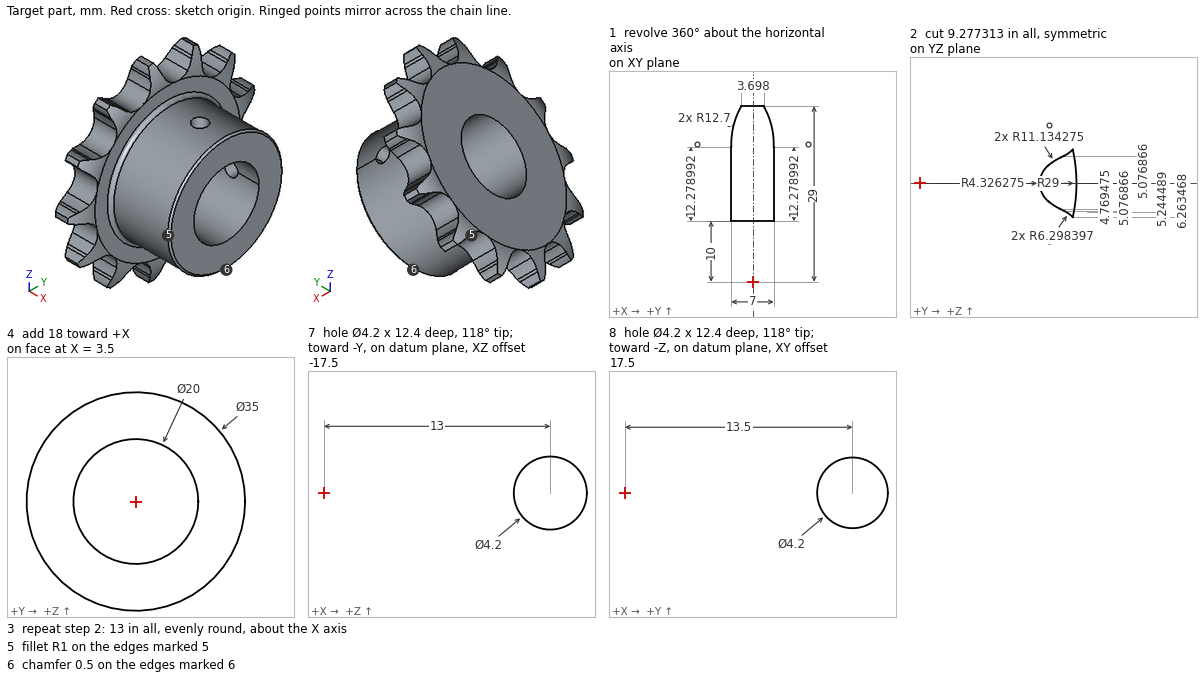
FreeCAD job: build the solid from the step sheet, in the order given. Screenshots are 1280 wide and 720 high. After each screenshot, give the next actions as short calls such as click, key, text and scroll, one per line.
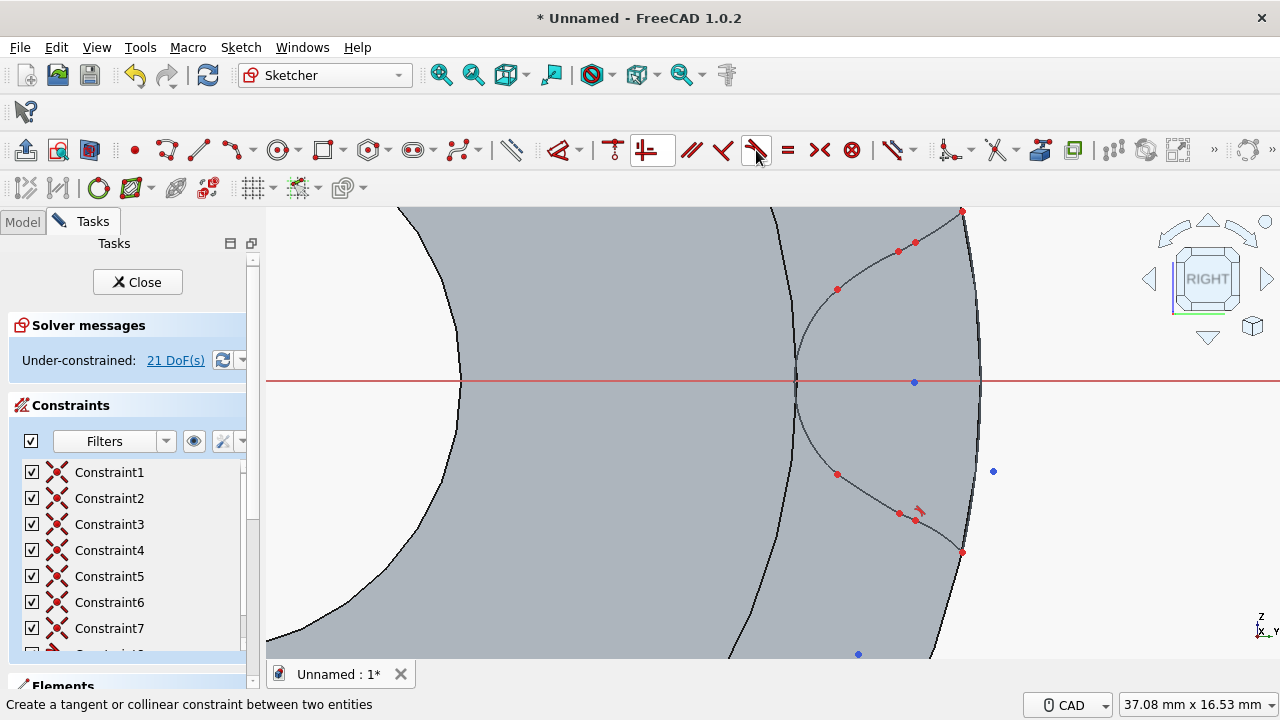
scroll(908, 517, up, 3)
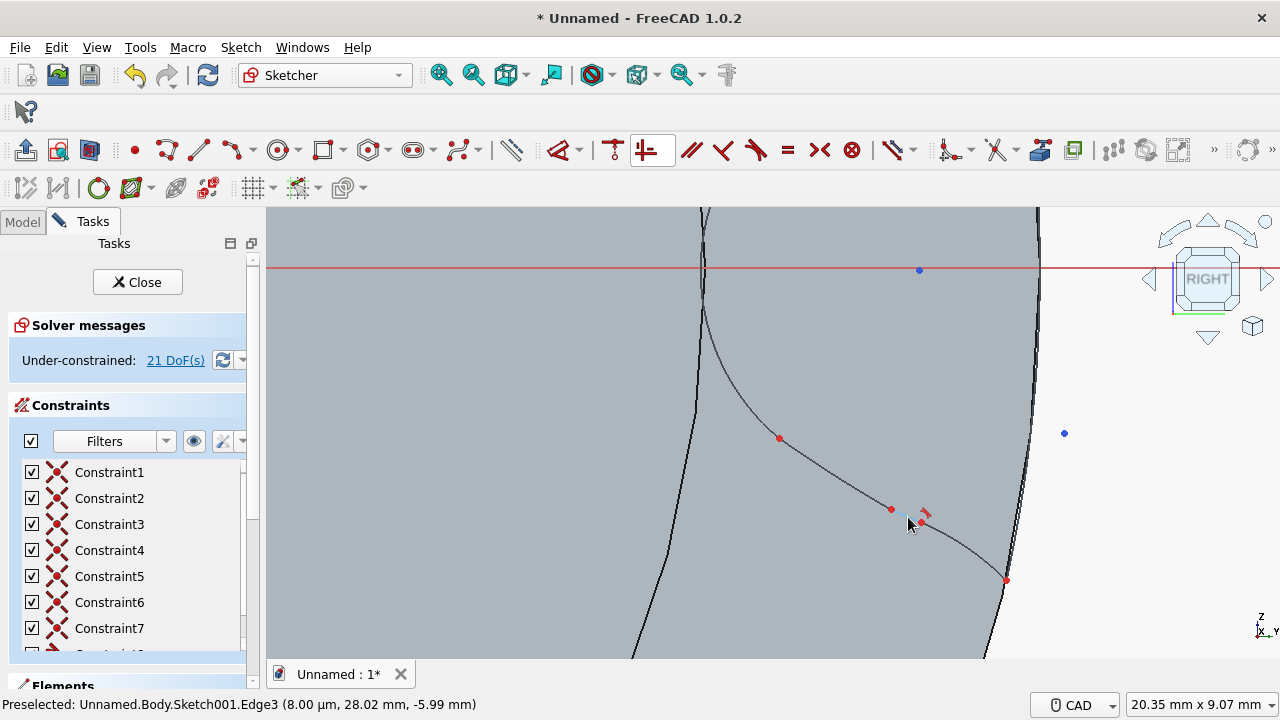
click(907, 516)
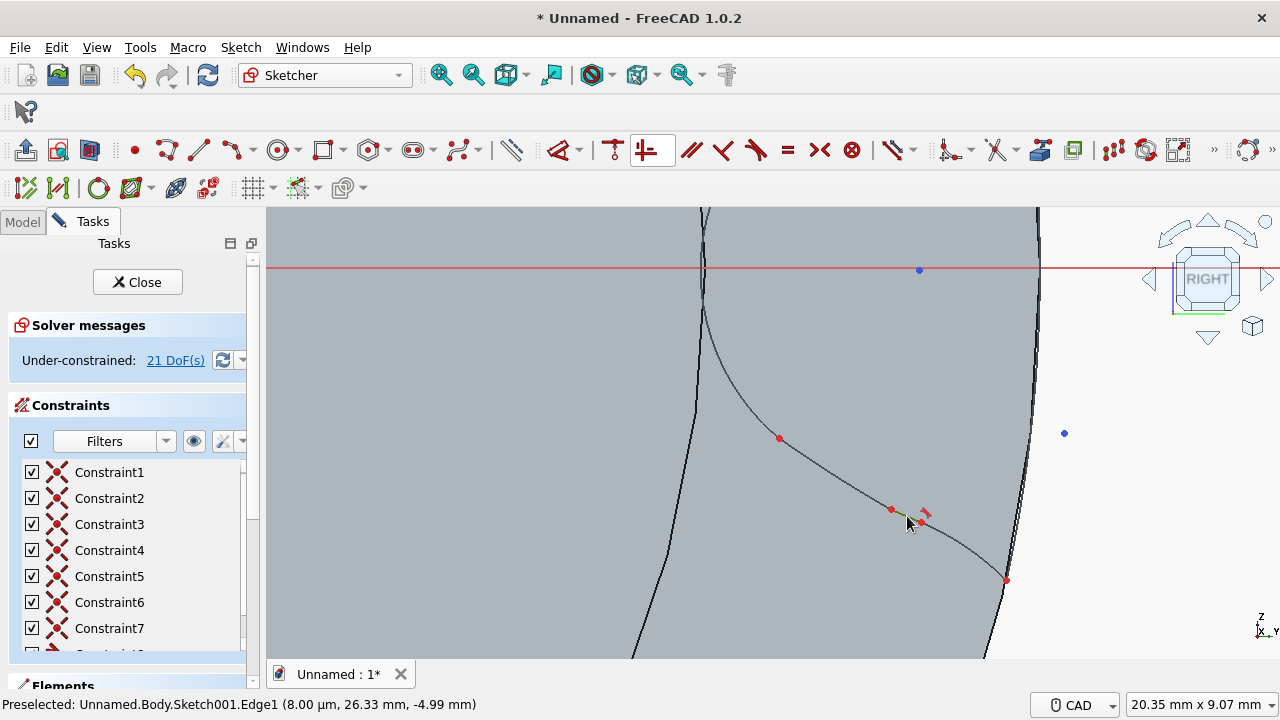
click(812, 461)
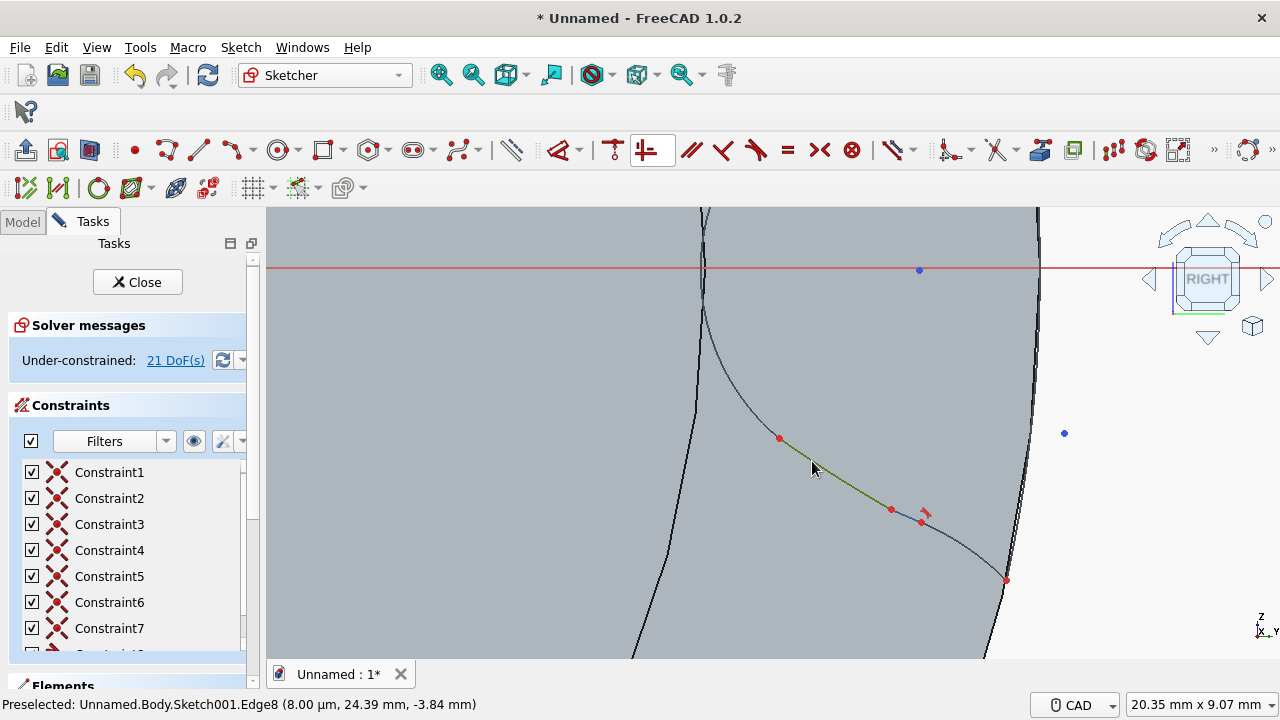
key(t)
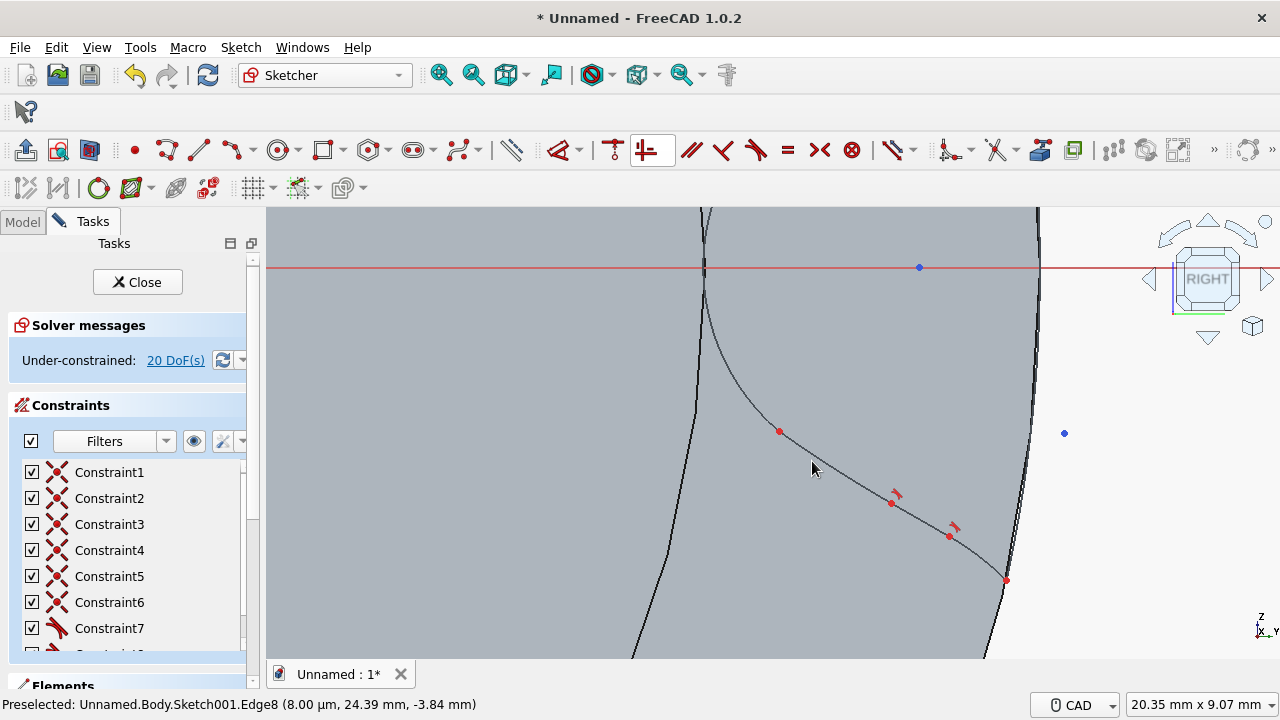
scroll(930, 529, down, 5)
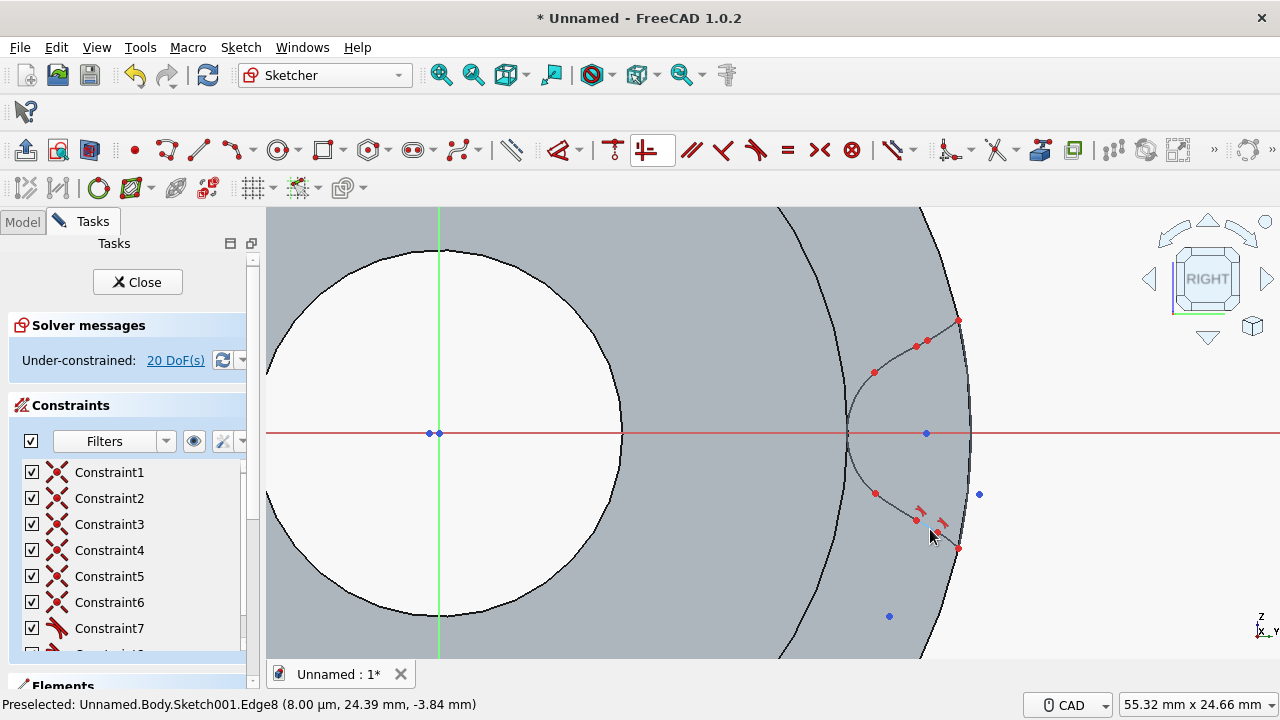
scroll(924, 343, up, 7)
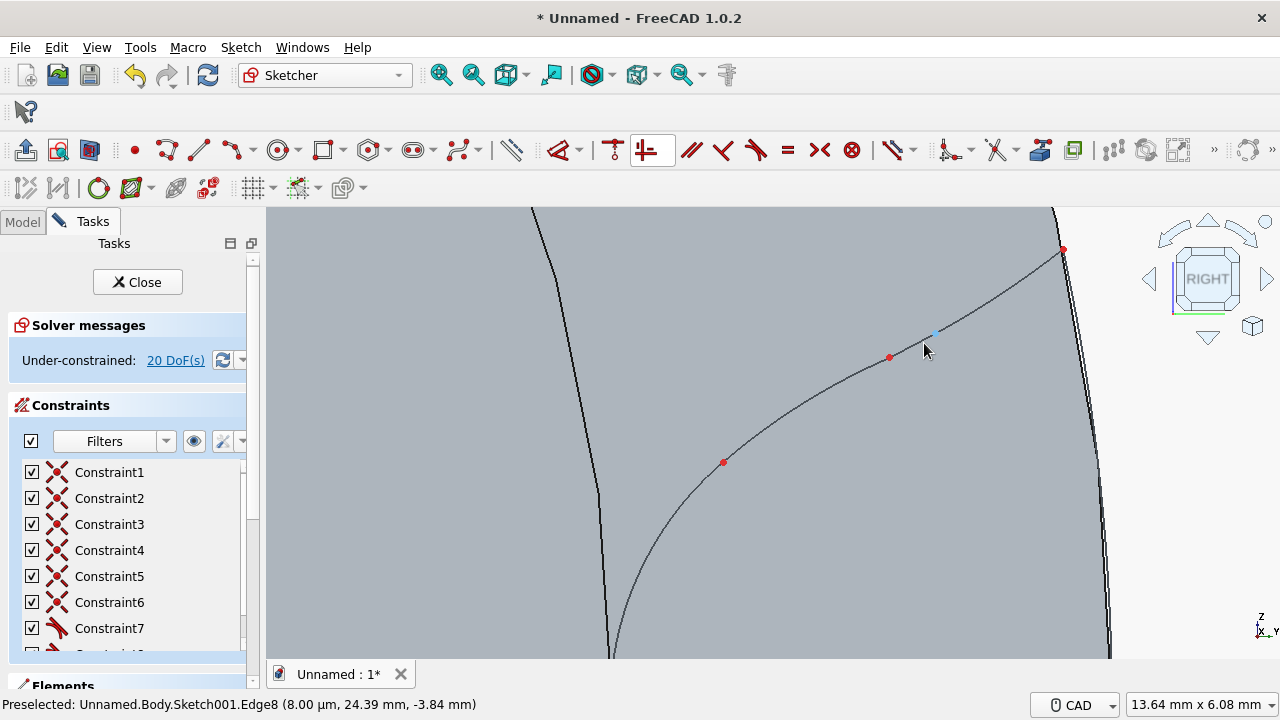
click(922, 341)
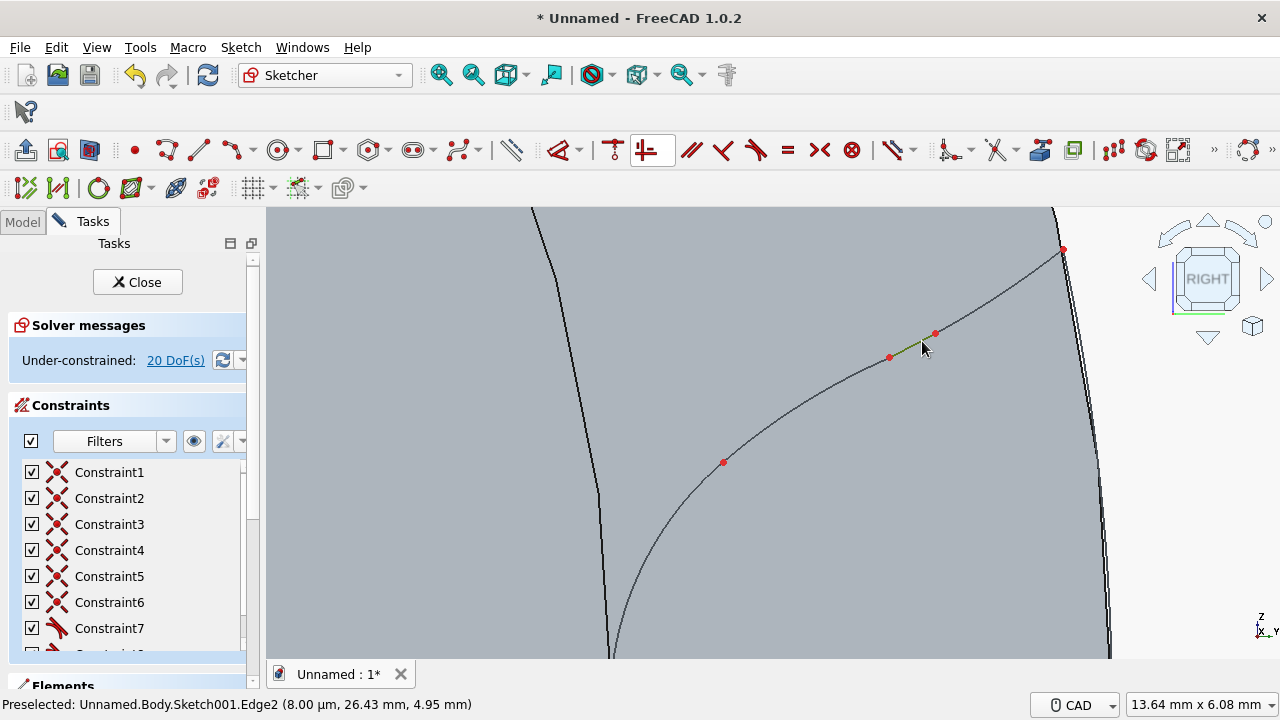
scroll(924, 343, down, 7)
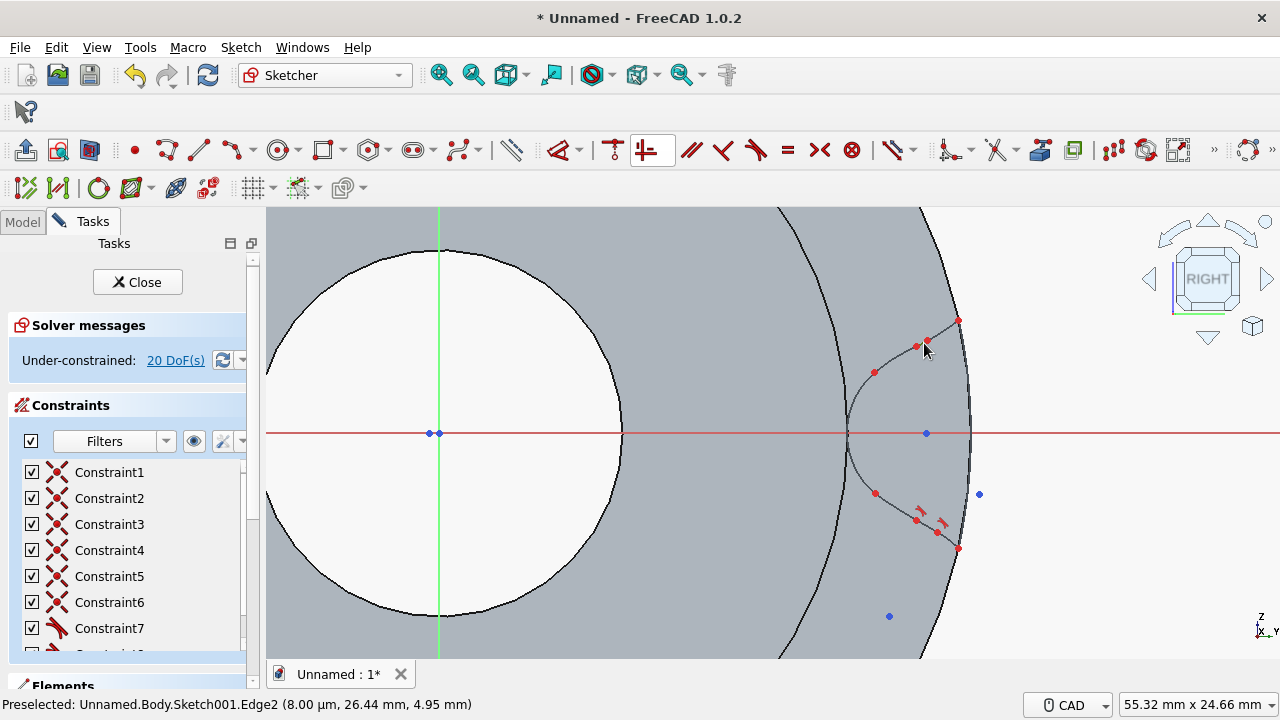
scroll(937, 335, up, 2)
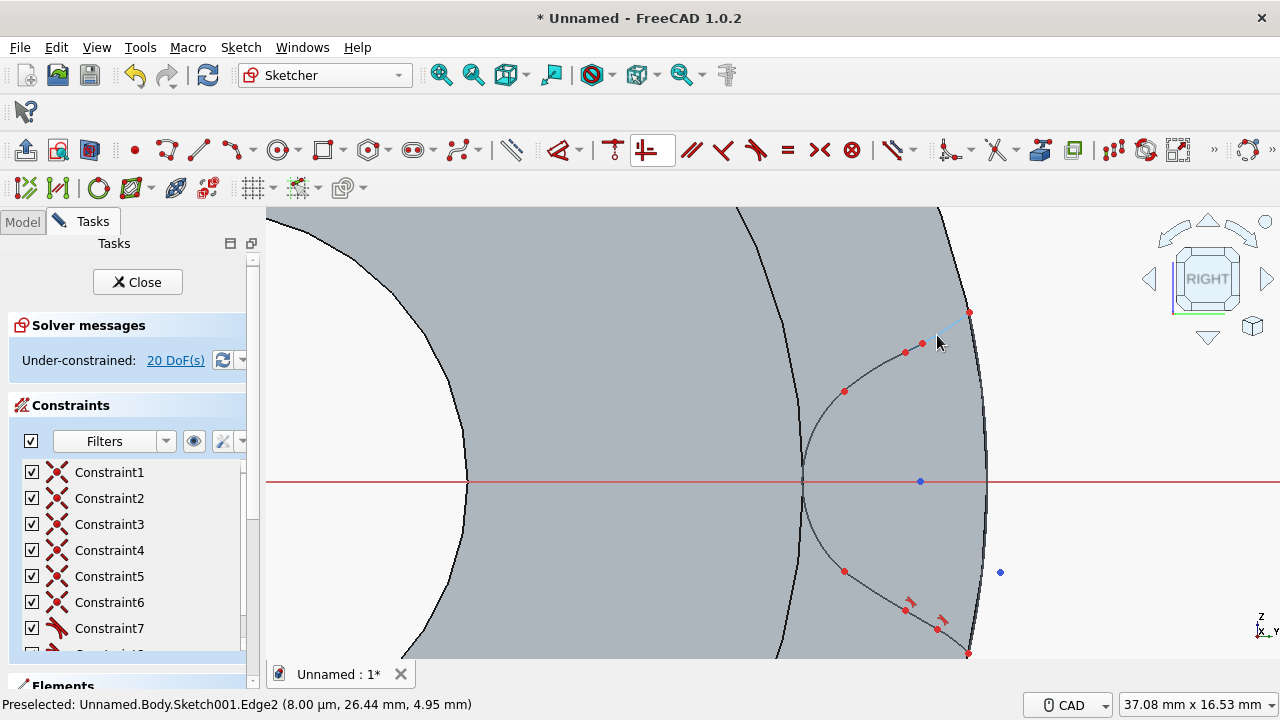
click(937, 335)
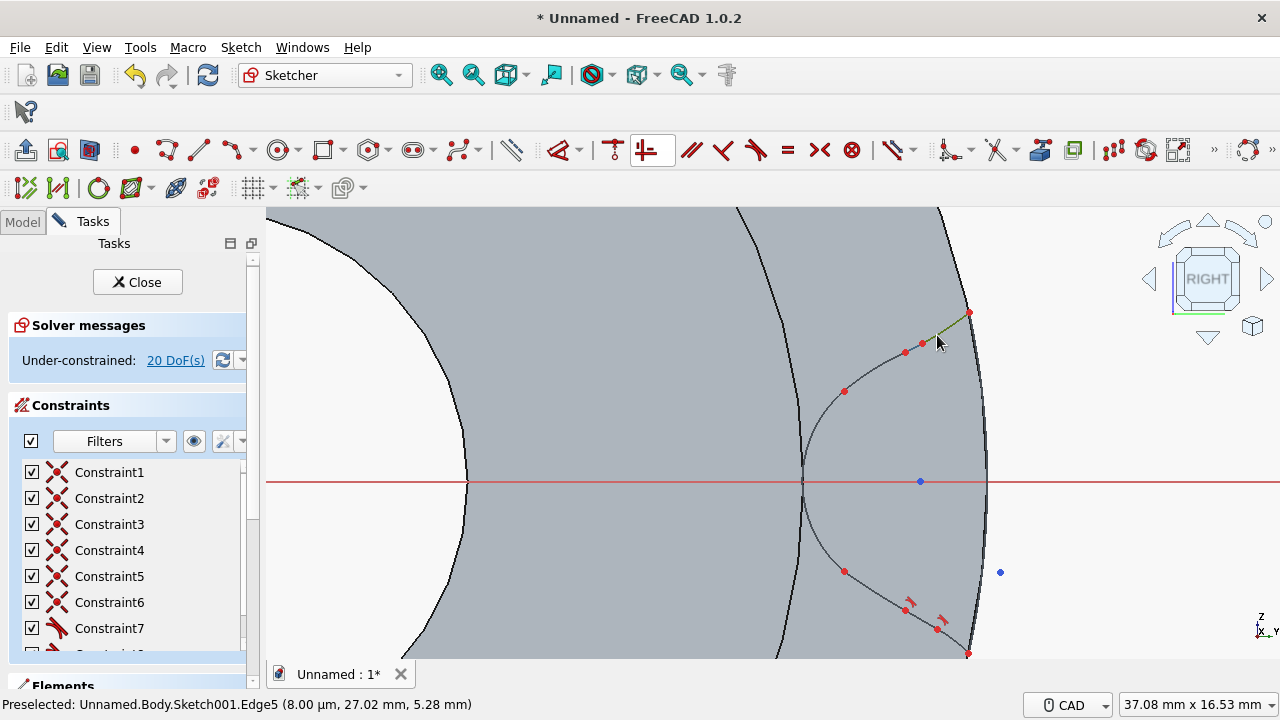
click(756, 150)